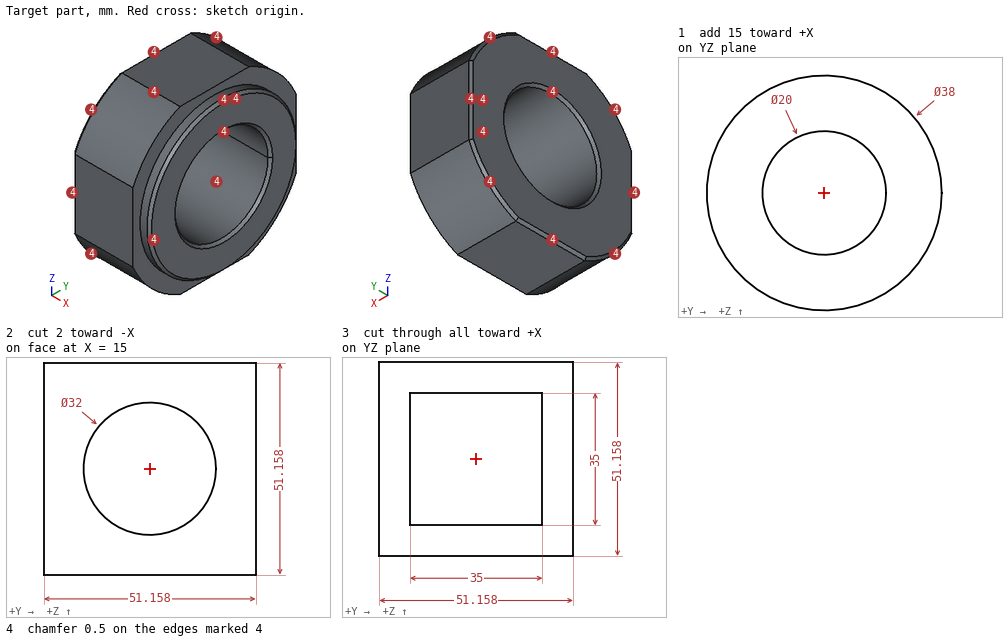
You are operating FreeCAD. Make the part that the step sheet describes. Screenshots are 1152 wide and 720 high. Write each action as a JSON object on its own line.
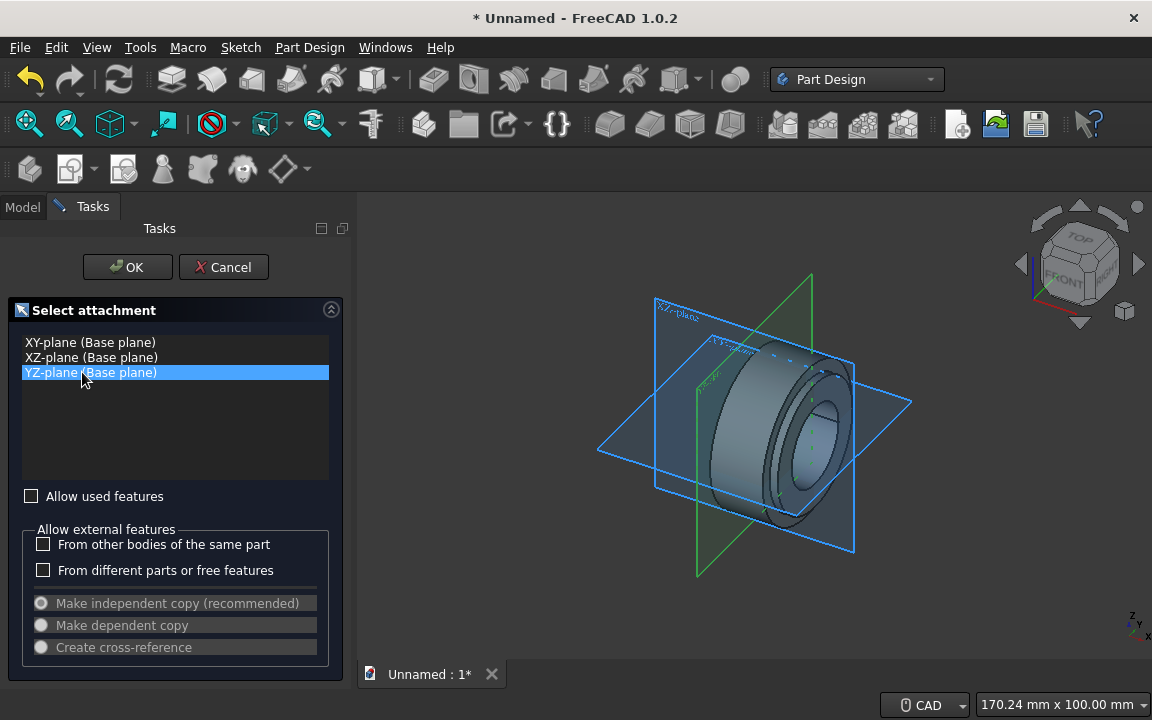
{"action": "left_click", "coordinate": [128, 267]}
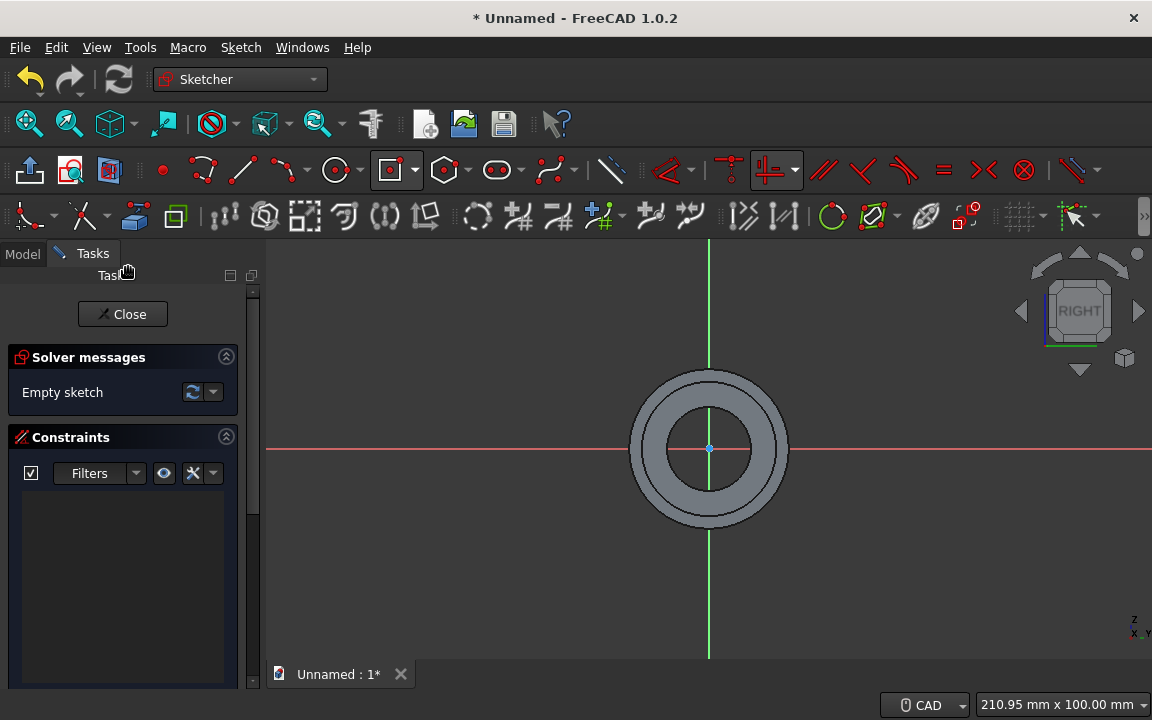
{"action": "key", "text": "q s"}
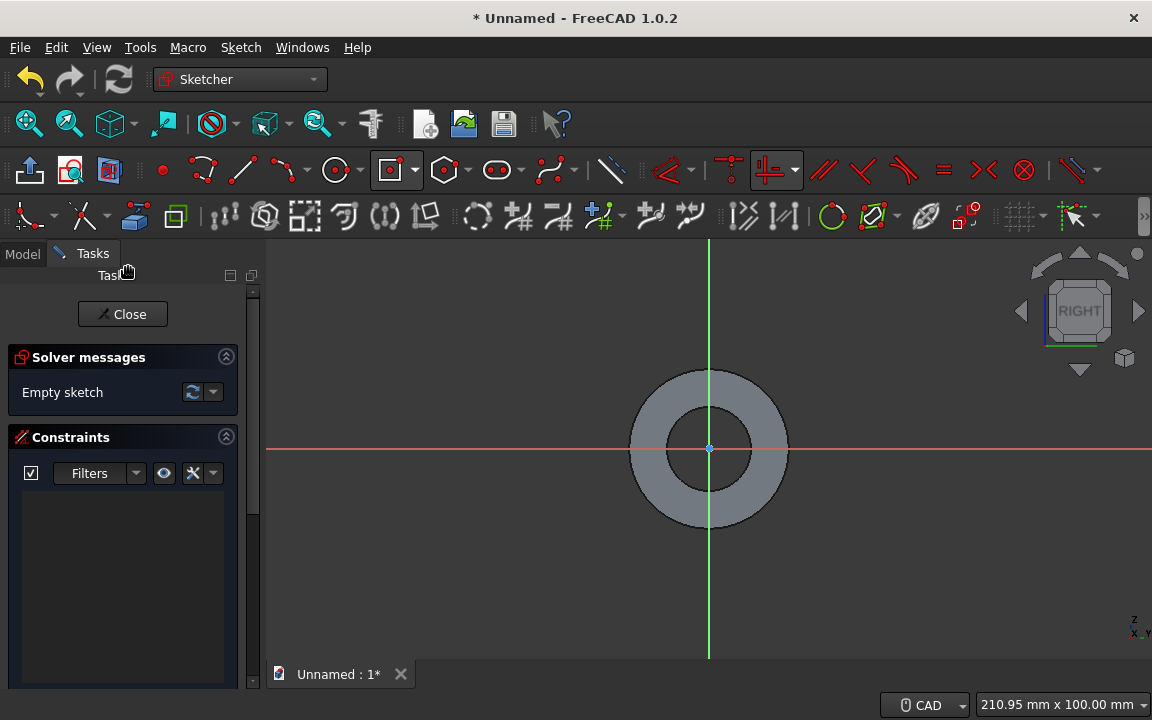
{"action": "left_click", "coordinate": [390, 170]}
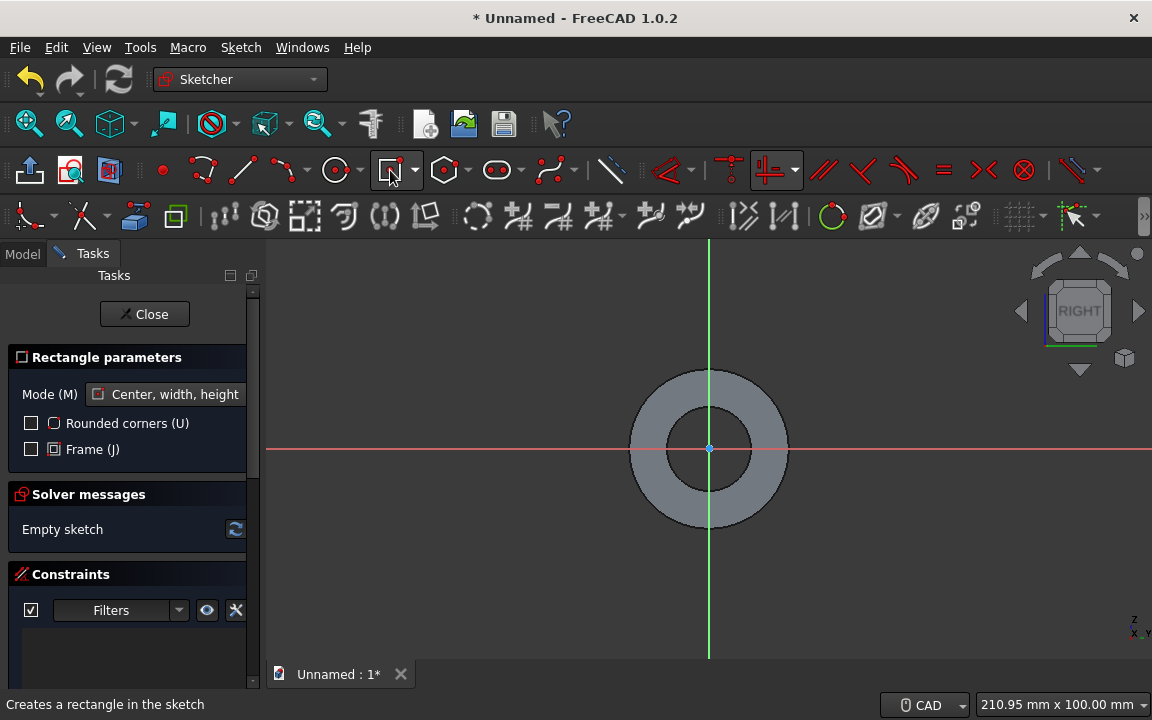
{"action": "left_click", "coordinate": [709, 449]}
{"action": "left_click", "coordinate": [816, 342]}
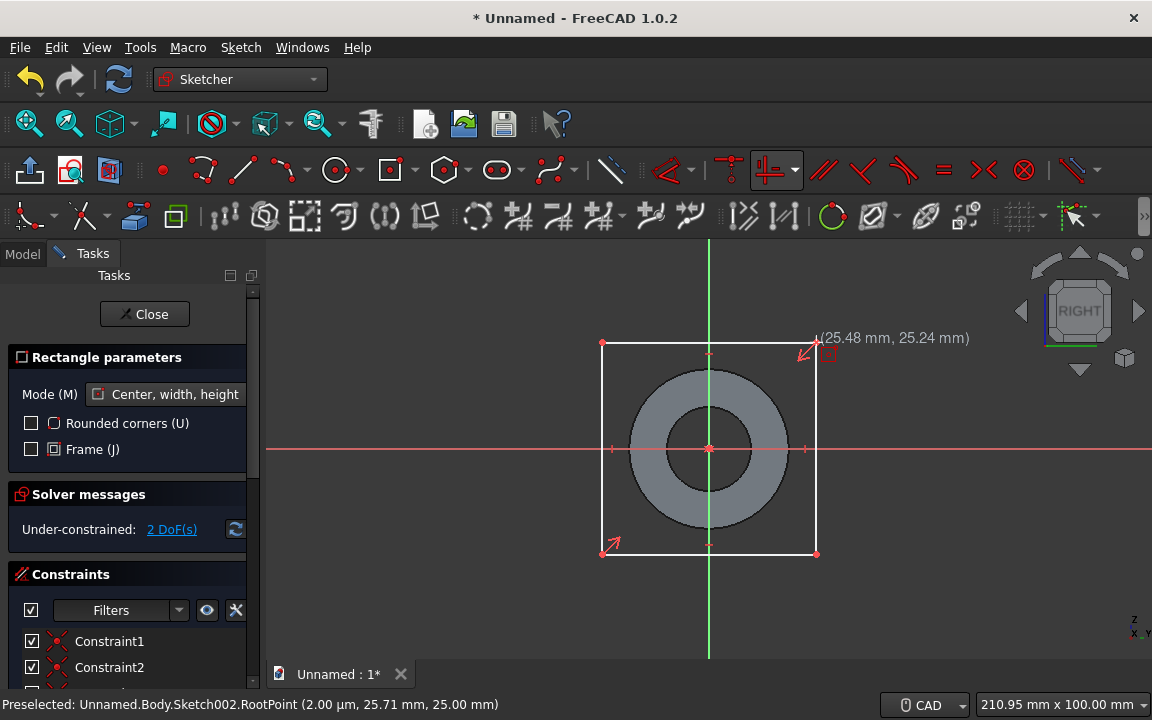
{"action": "left_click", "coordinate": [709, 449]}
{"action": "left_click", "coordinate": [782, 376]}
{"action": "key", "text": "Escape"}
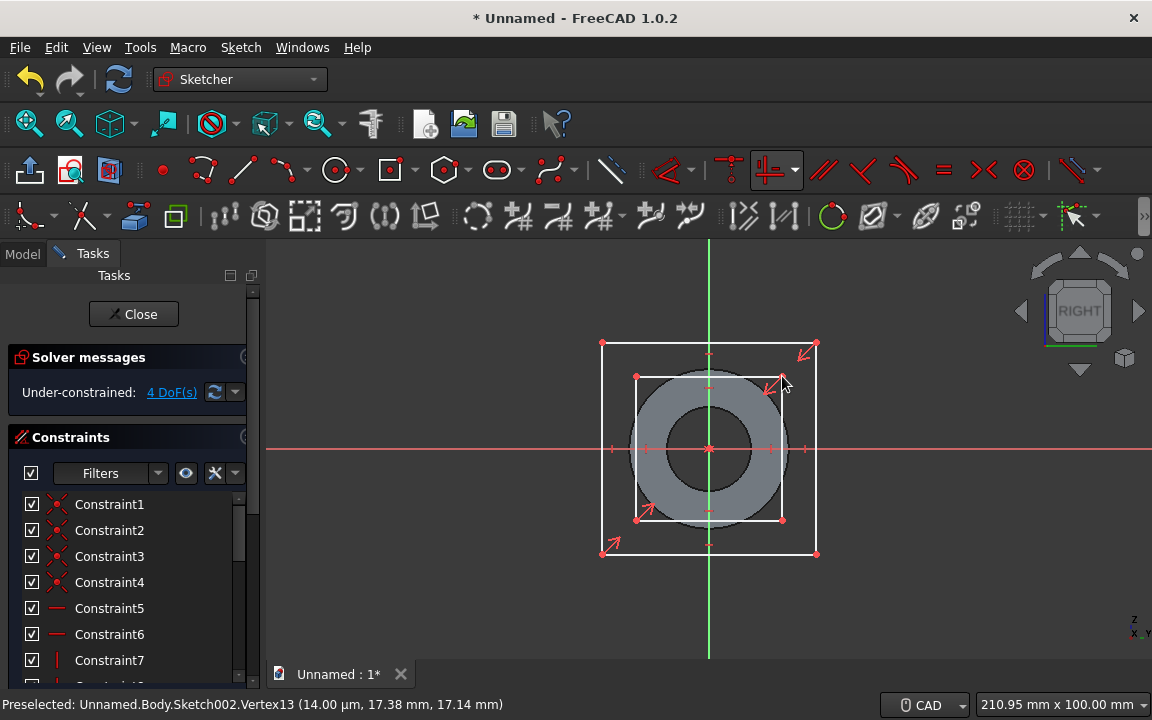
{"action": "key", "text": "d"}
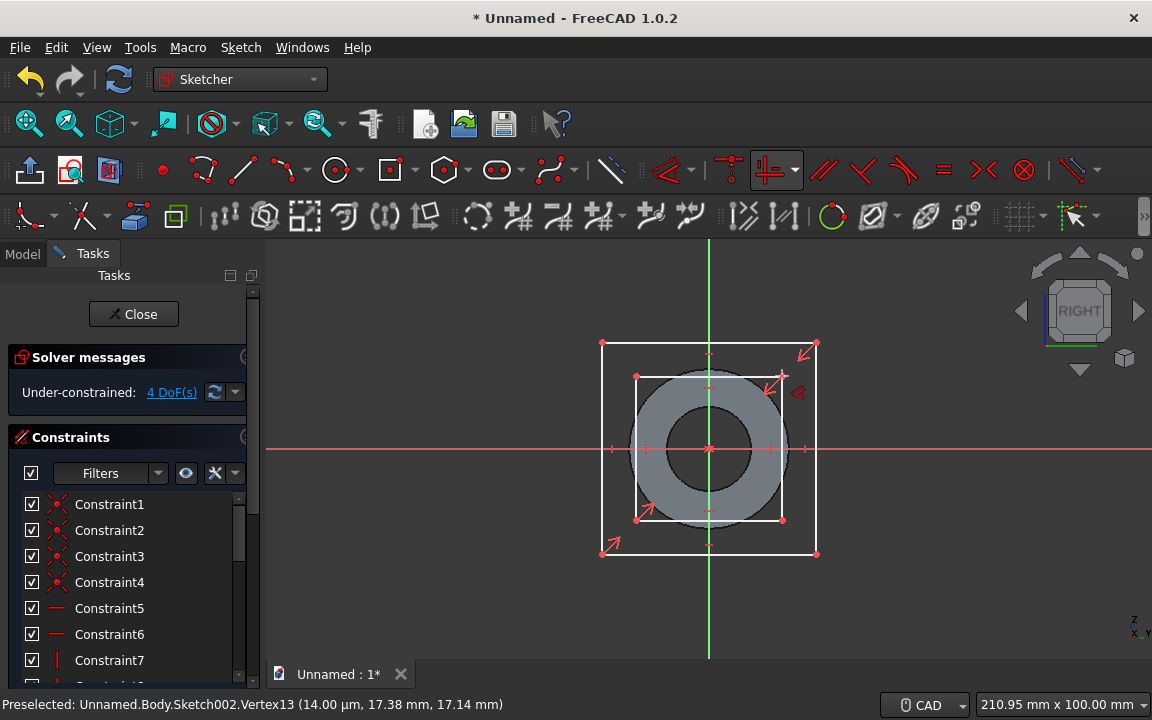
{"action": "left_click", "coordinate": [680, 521]}
{"action": "left_click", "coordinate": [675, 487]}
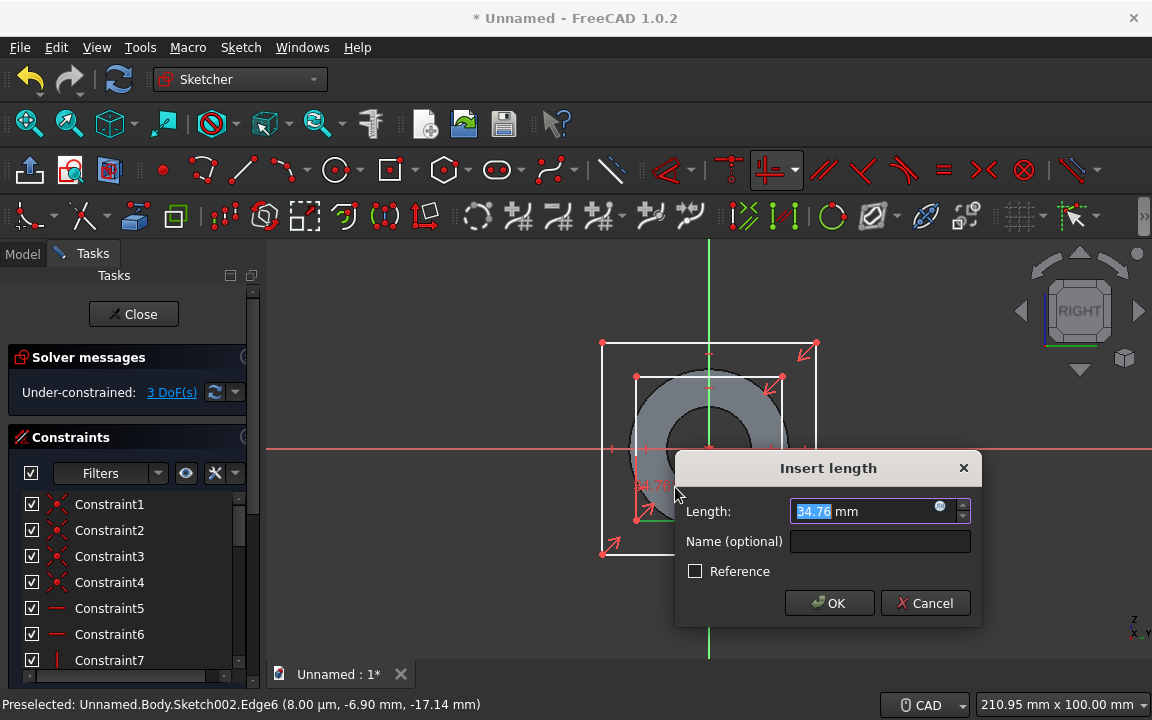
{"action": "type", "text": "35"}
{"action": "key", "text": "Return"}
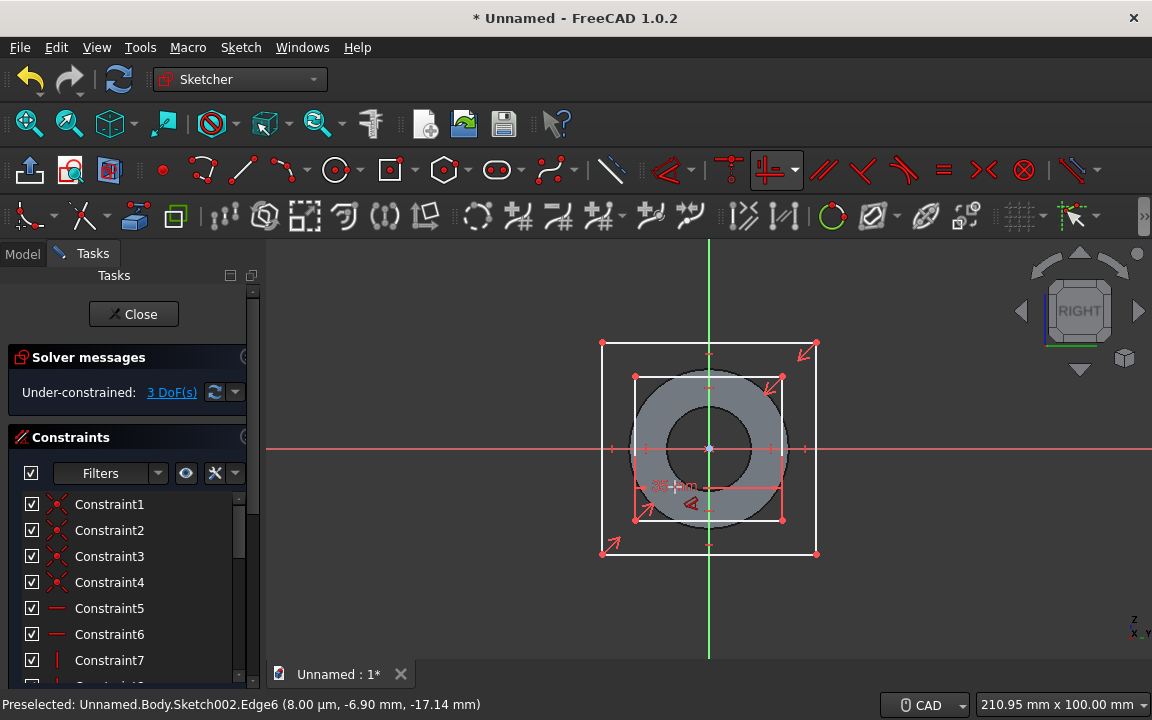
{"action": "left_click", "coordinate": [782, 478]}
{"action": "left_click", "coordinate": [748, 416]}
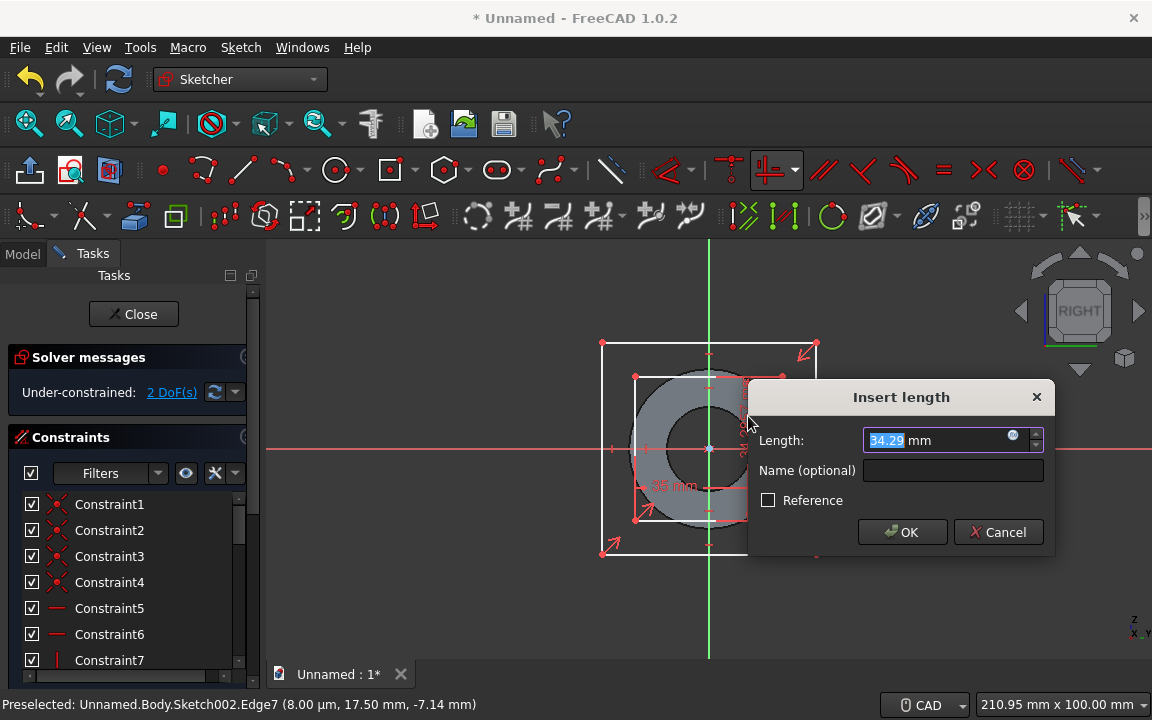
{"action": "type", "text": "35"}
{"action": "key", "text": "Return"}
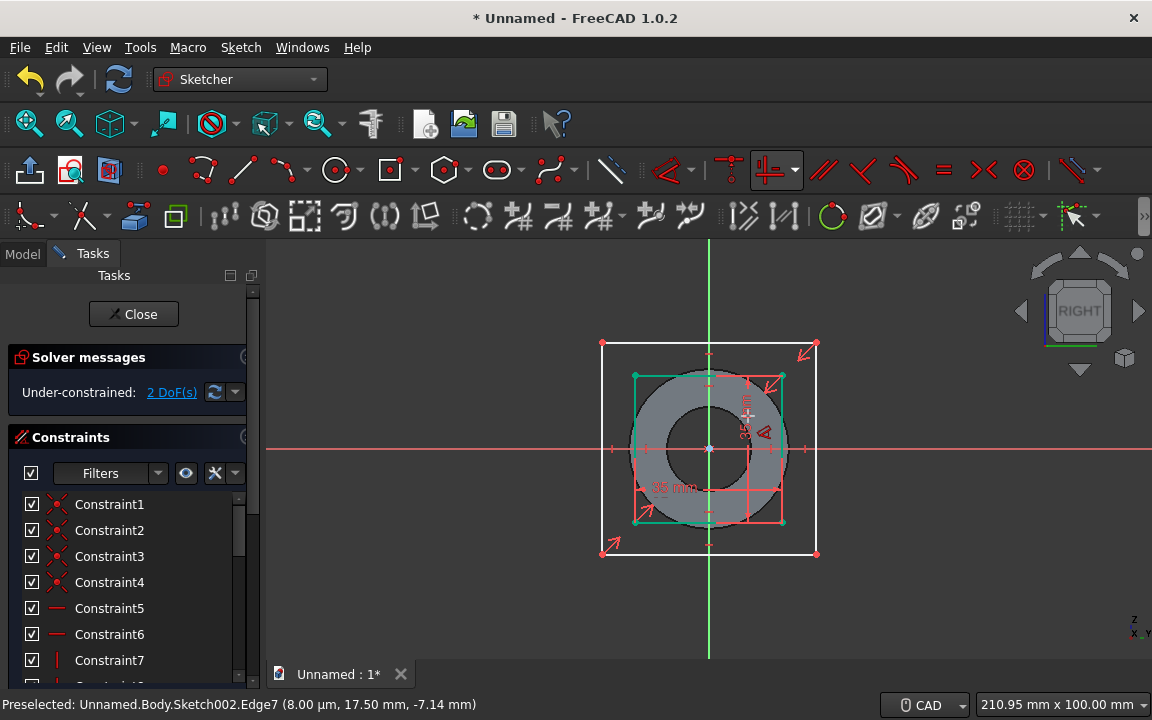
{"action": "left_click", "coordinate": [666, 555]}
{"action": "left_click", "coordinate": [660, 589]}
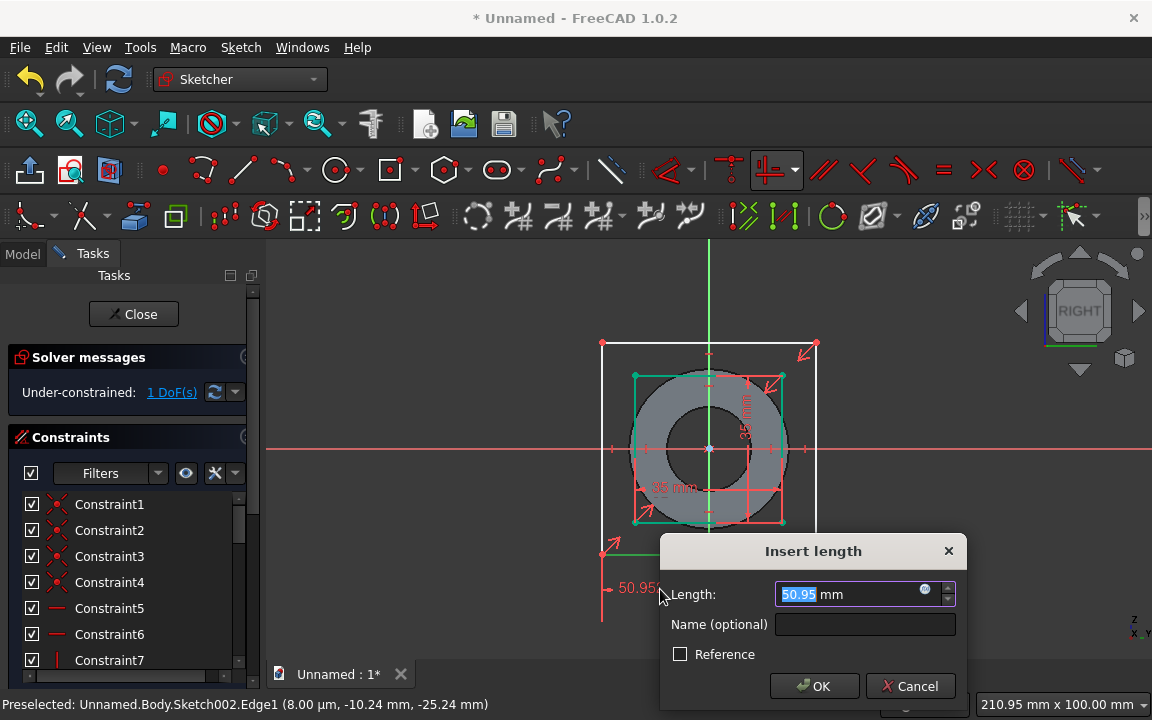
{"action": "type", "text": "51.158"}
{"action": "key", "text": "Return"}